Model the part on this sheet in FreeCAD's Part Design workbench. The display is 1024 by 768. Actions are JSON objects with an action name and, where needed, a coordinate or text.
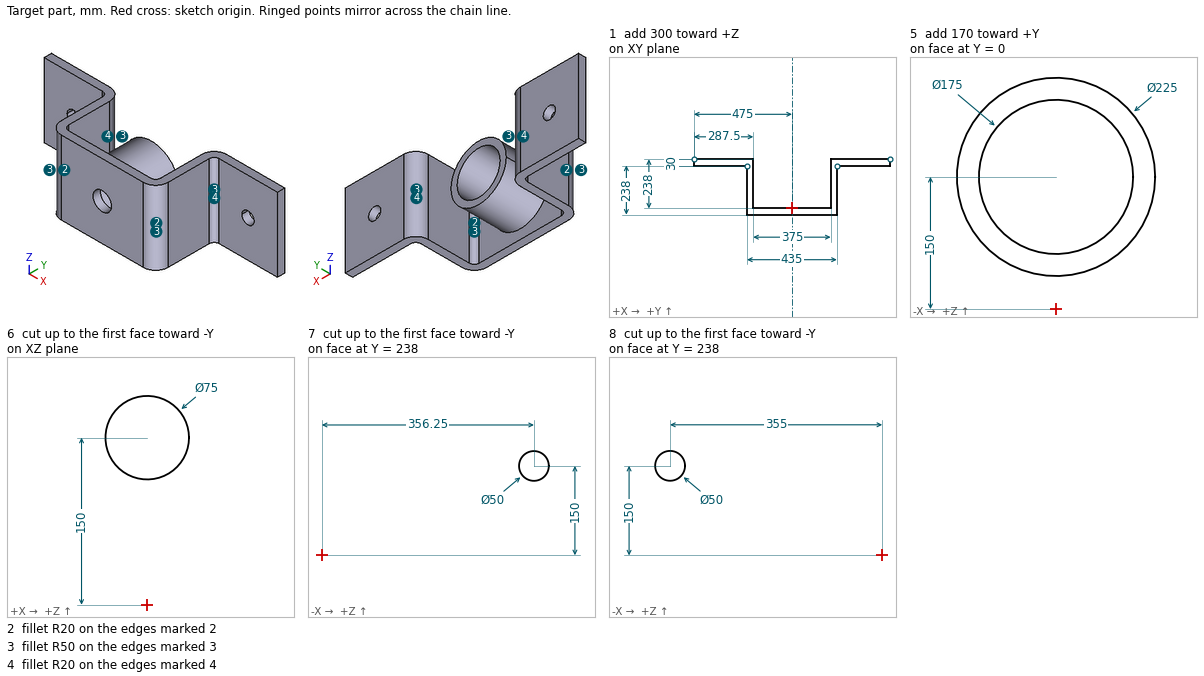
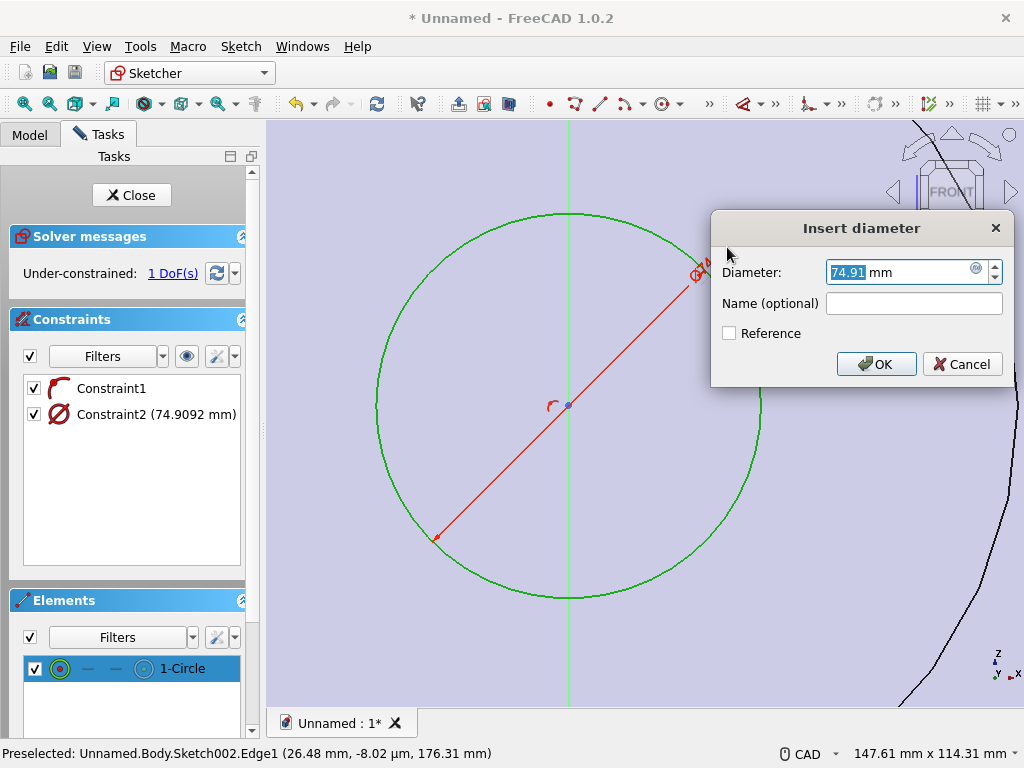
{"action": "type", "text": "75"}
{"action": "key", "text": "Return"}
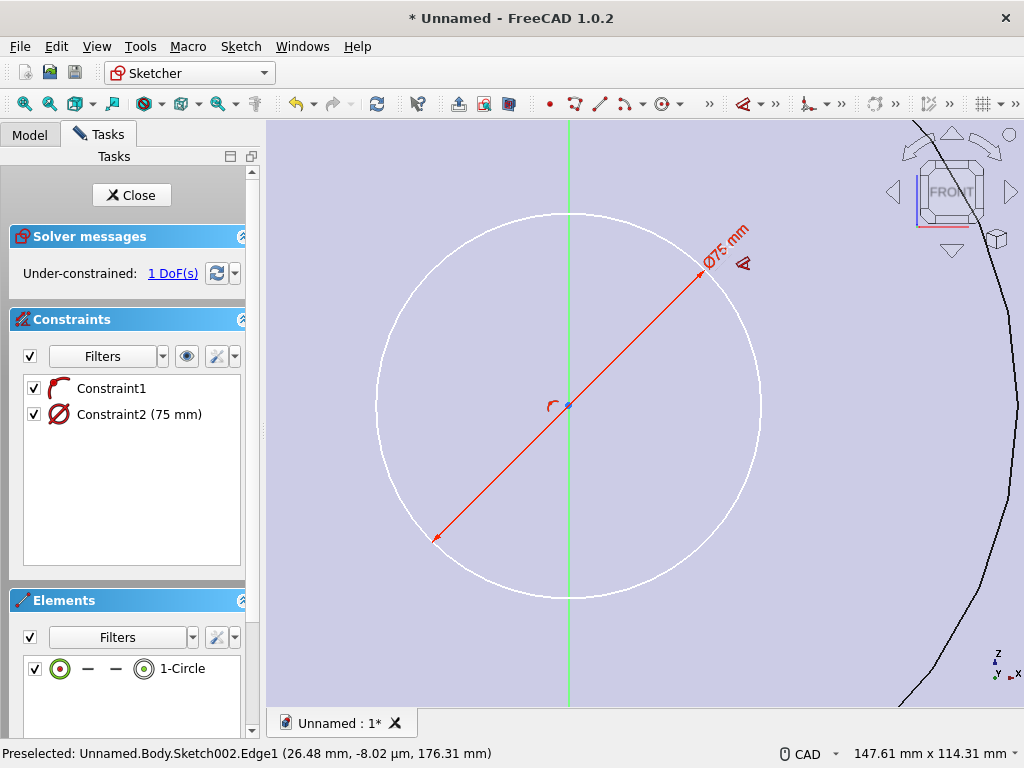
{"action": "left_click", "coordinate": [569, 406]}
{"action": "left_click", "coordinate": [603, 542]}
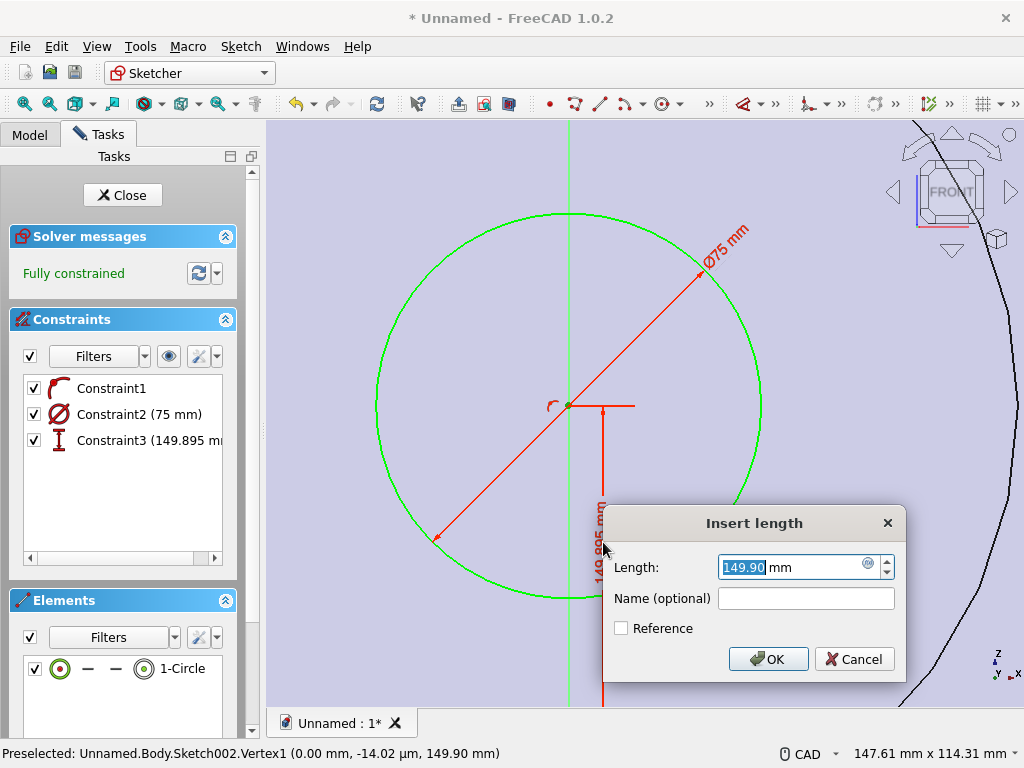
{"action": "type", "text": "150"}
{"action": "key", "text": "Return"}
{"action": "key", "text": "Escape"}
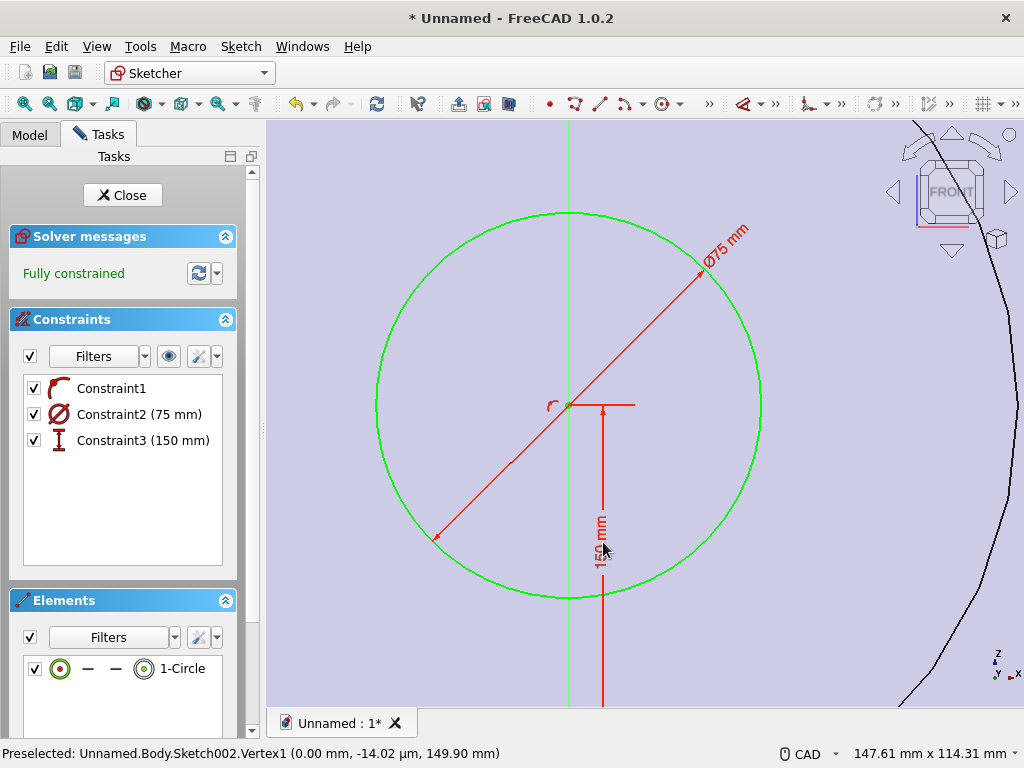
{"action": "left_click", "coordinate": [123, 195]}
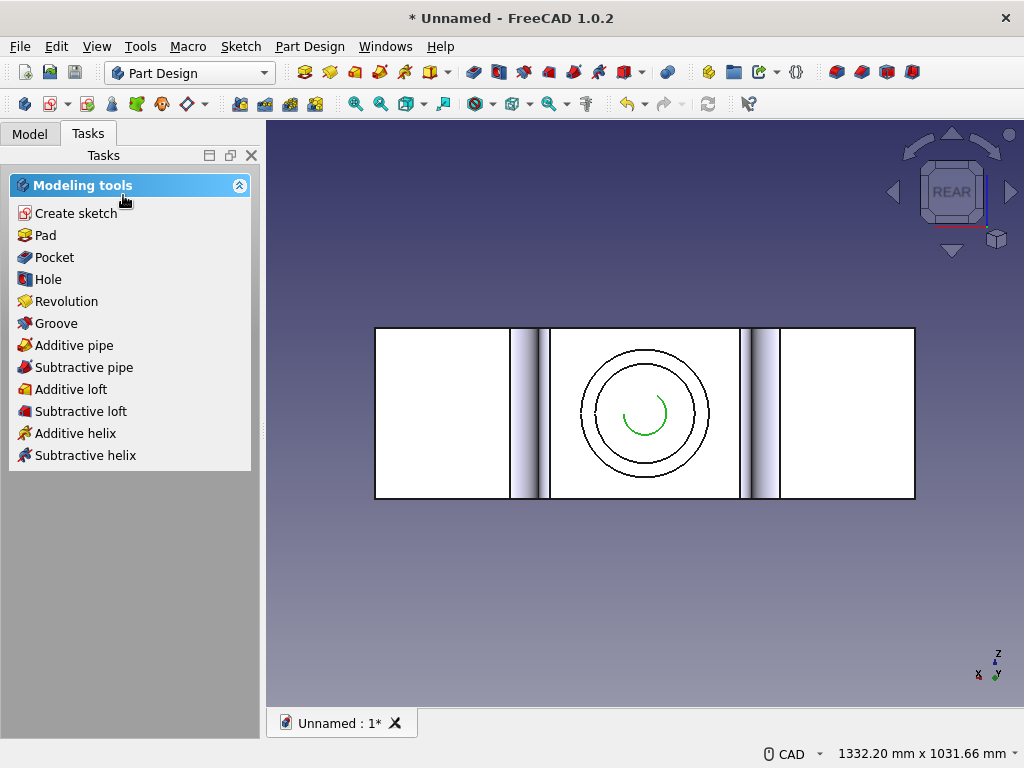
{"action": "left_click", "coordinate": [474, 72]}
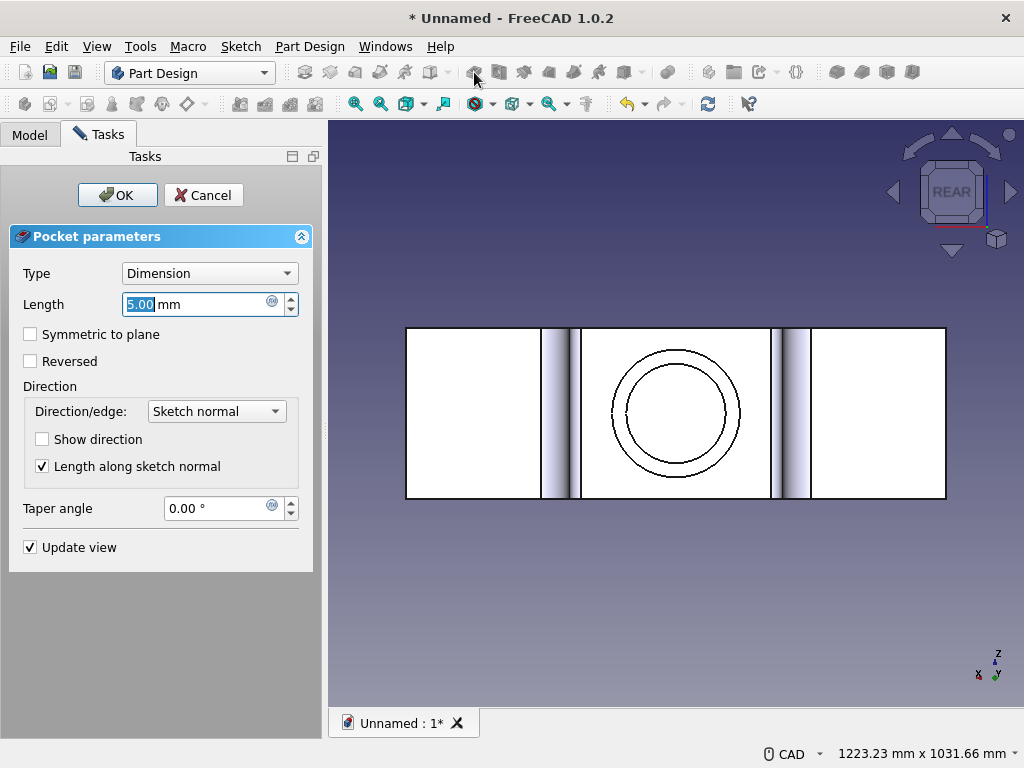
{"action": "left_click", "coordinate": [210, 274]}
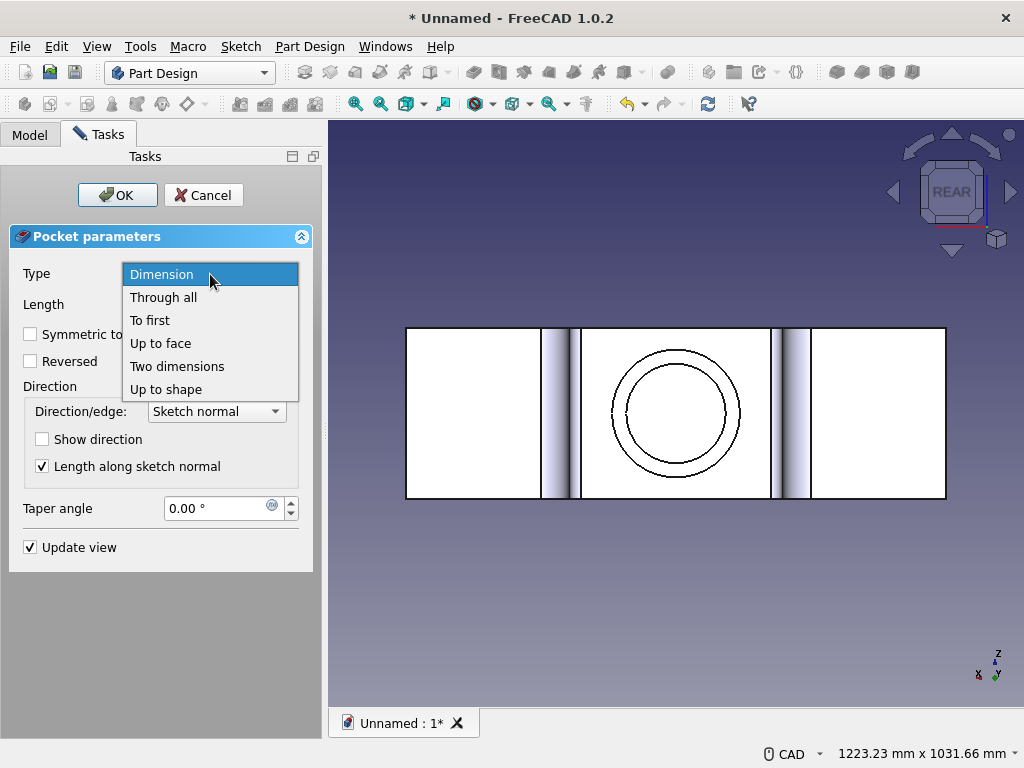
{"action": "left_click", "coordinate": [208, 320]}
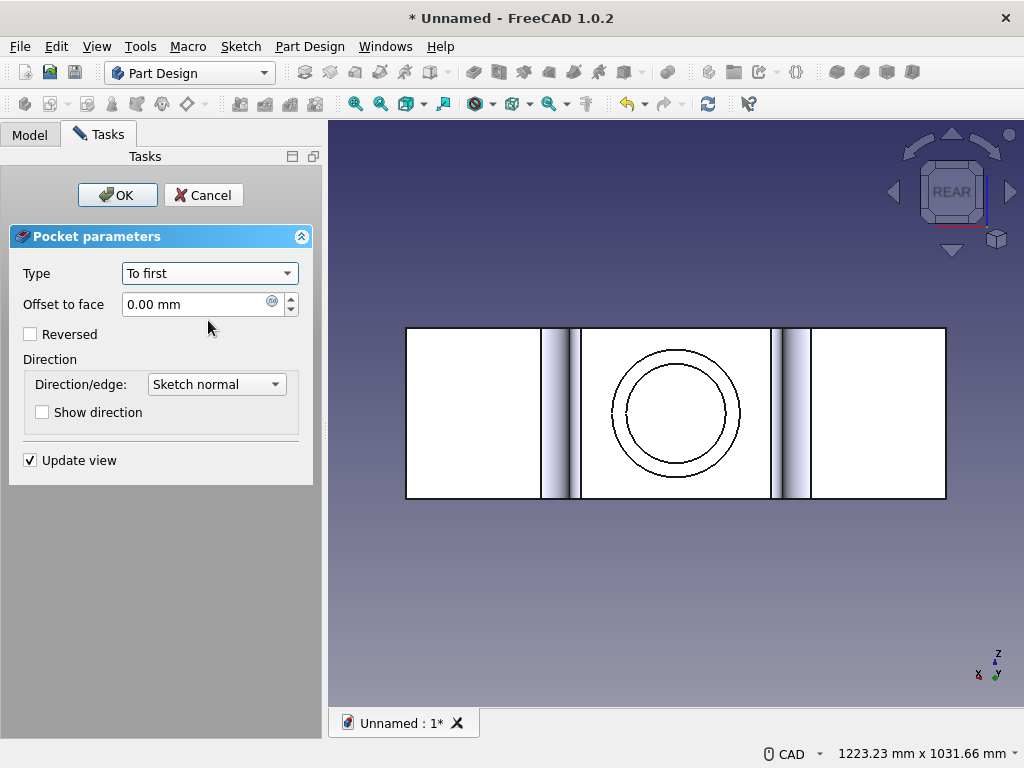
{"action": "left_click", "coordinate": [31, 334]}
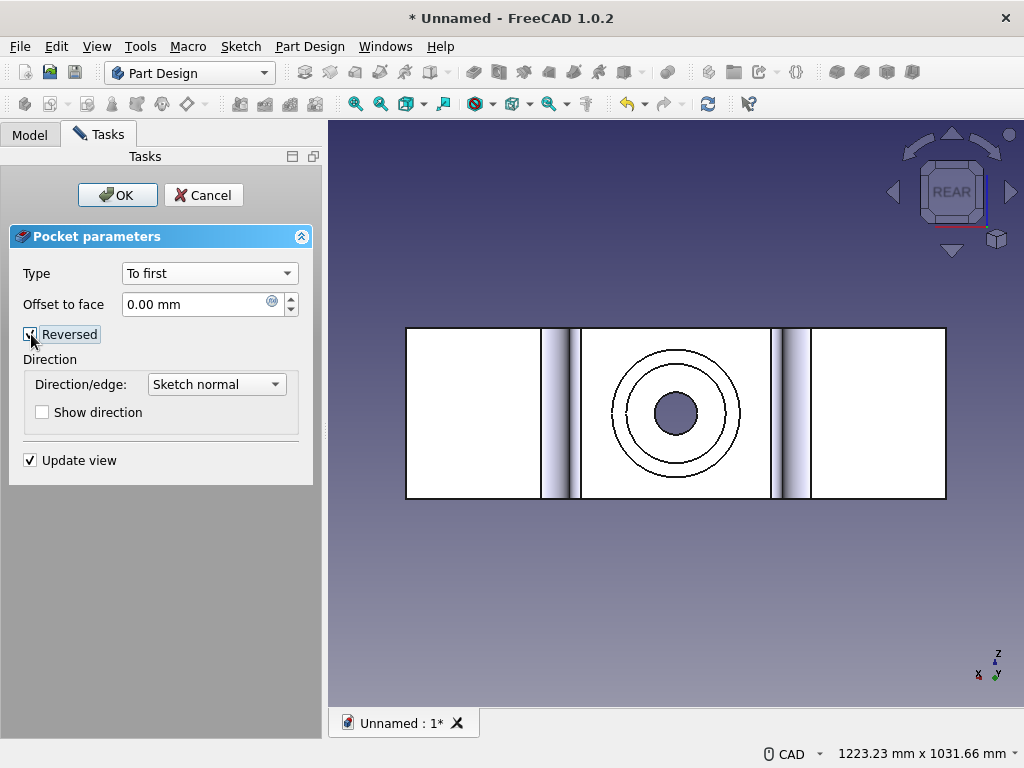
{"action": "left_click", "coordinate": [118, 195]}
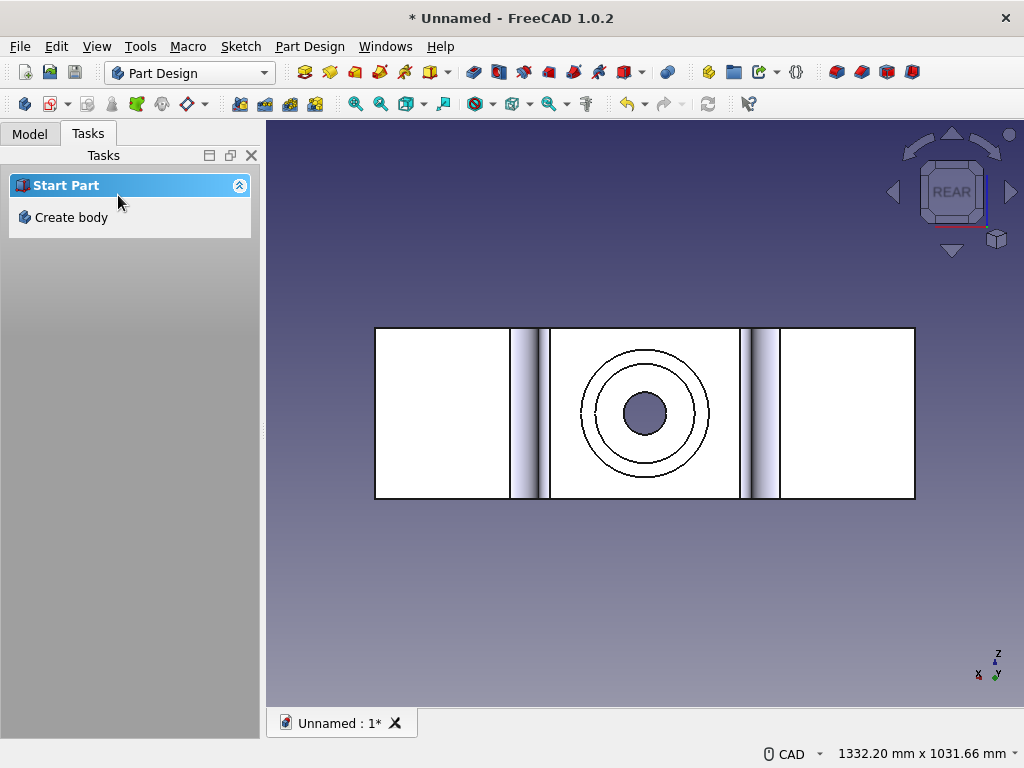
{"action": "left_click", "coordinate": [442, 412]}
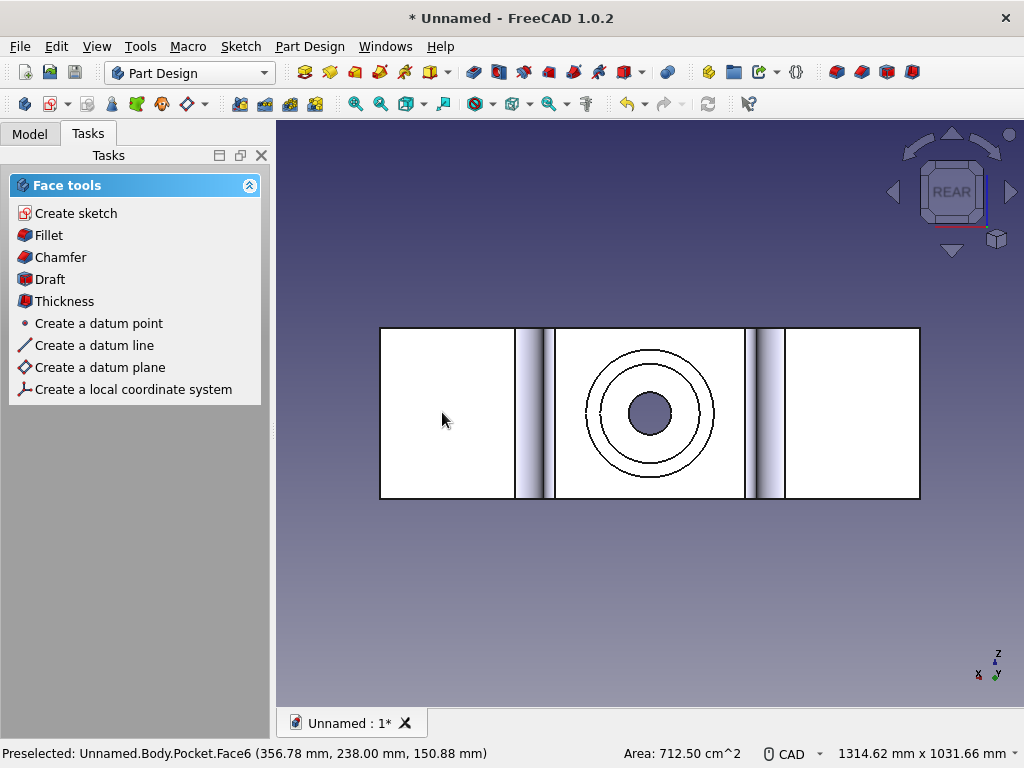
{"action": "left_click", "coordinate": [50, 104]}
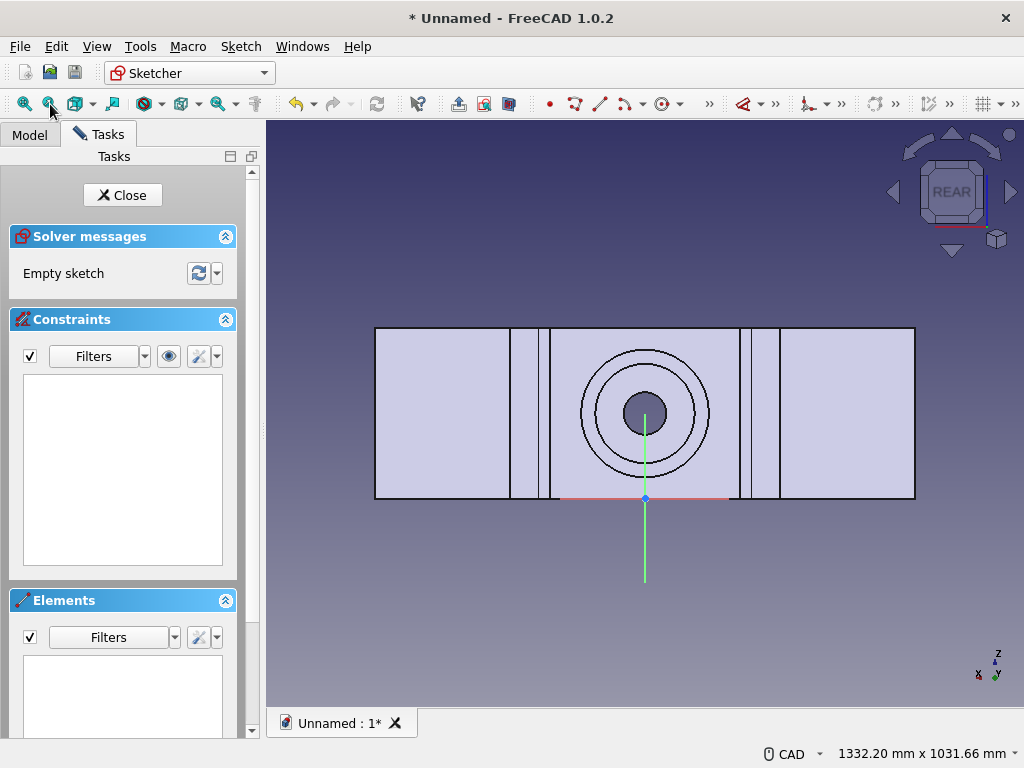
{"action": "scroll", "coordinate": [576, 414], "scroll_direction": "down", "scroll_amount": 5}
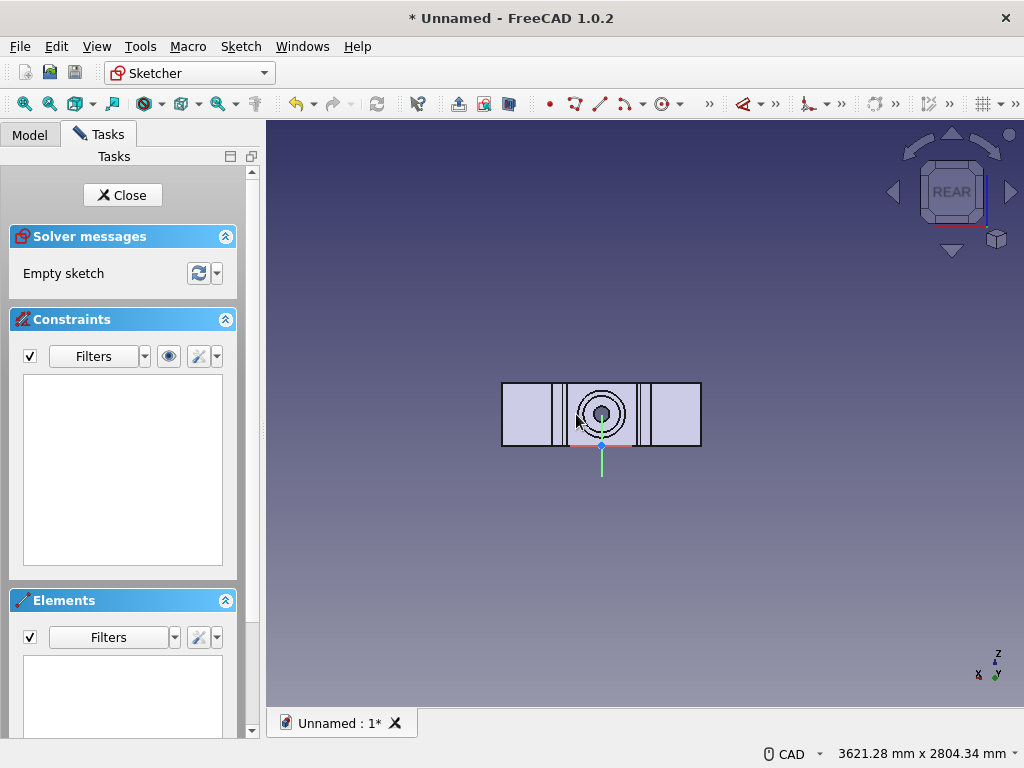
{"action": "scroll", "coordinate": [681, 414], "scroll_direction": "up", "scroll_amount": 15}